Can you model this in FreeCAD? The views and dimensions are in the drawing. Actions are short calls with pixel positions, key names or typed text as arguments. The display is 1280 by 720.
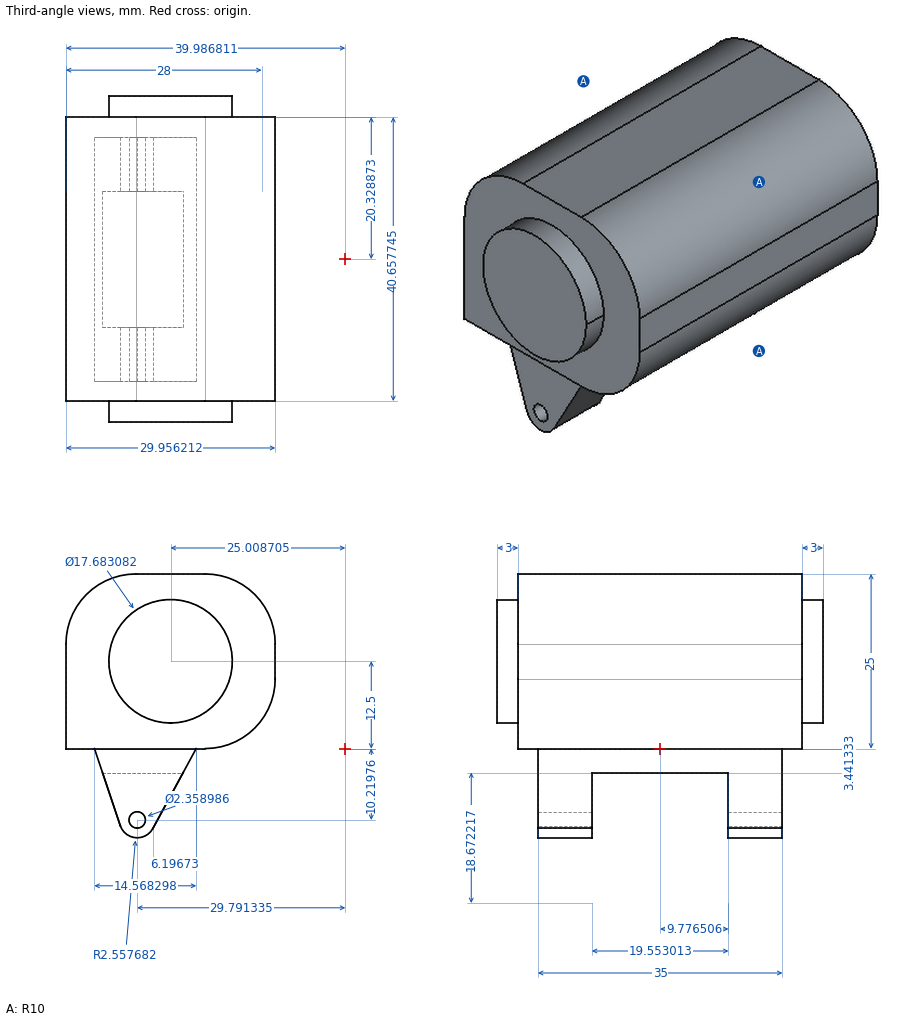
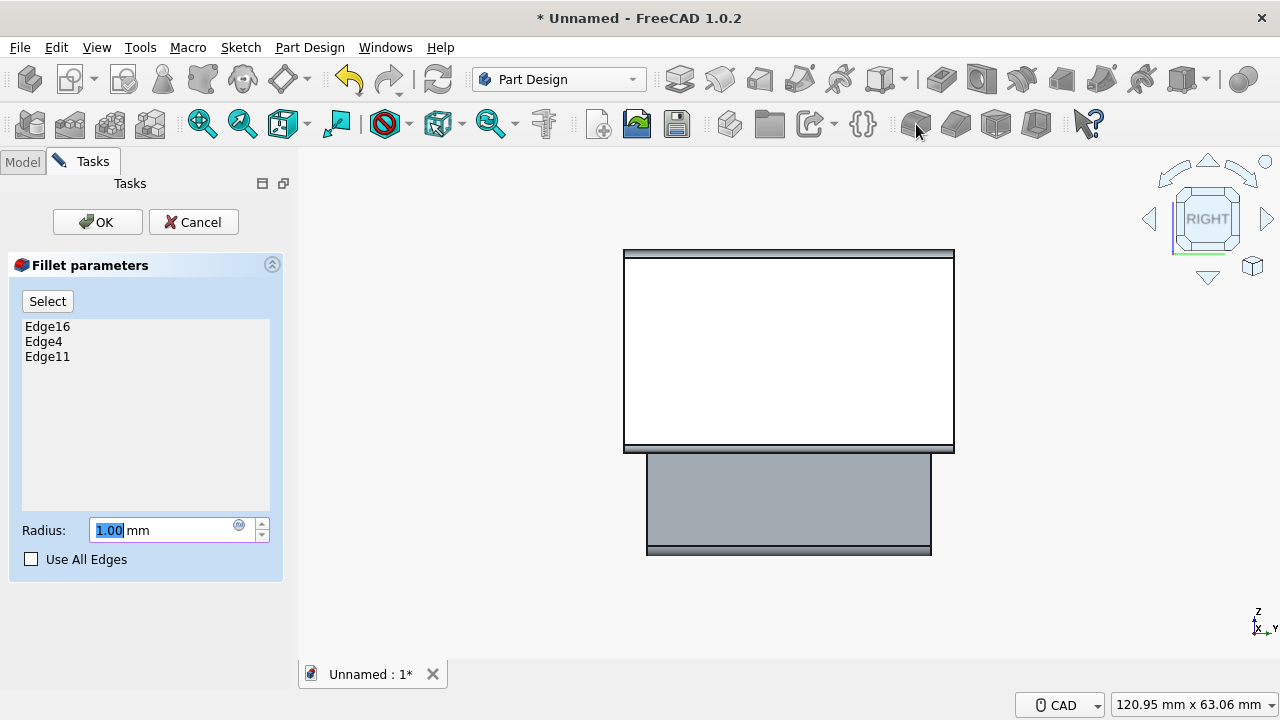
text(10)
key(Tab)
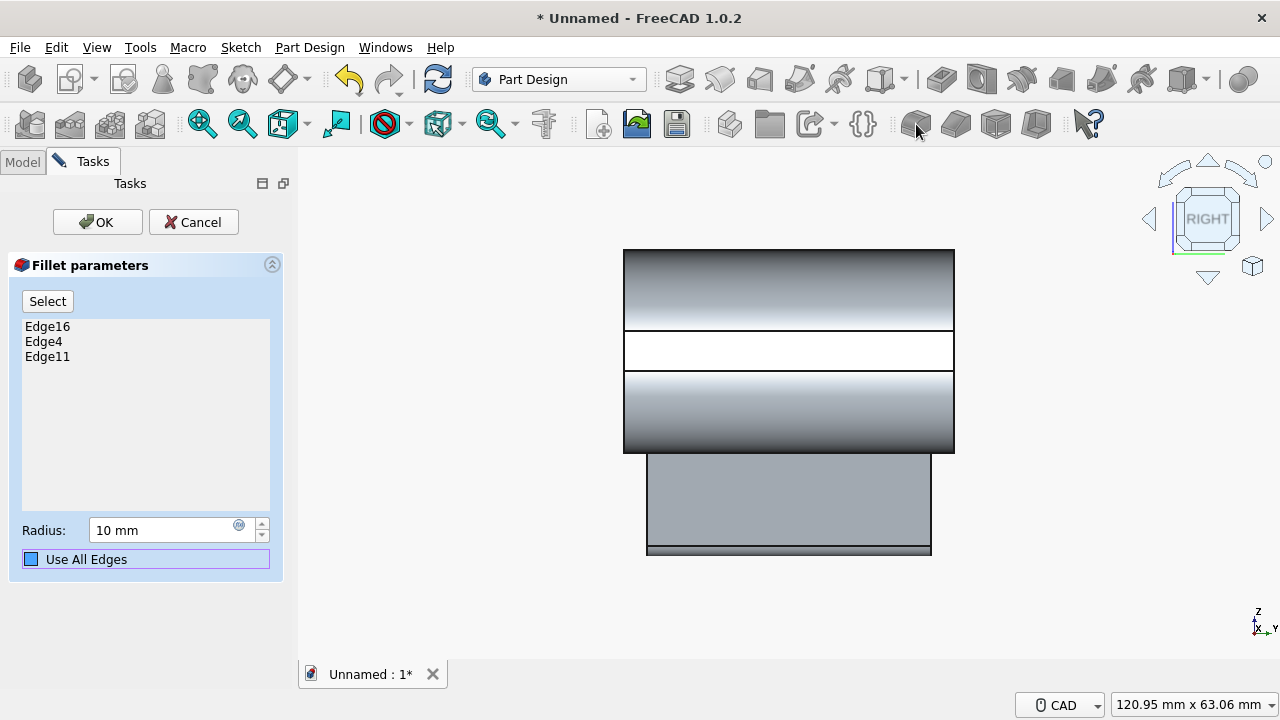
click(98, 222)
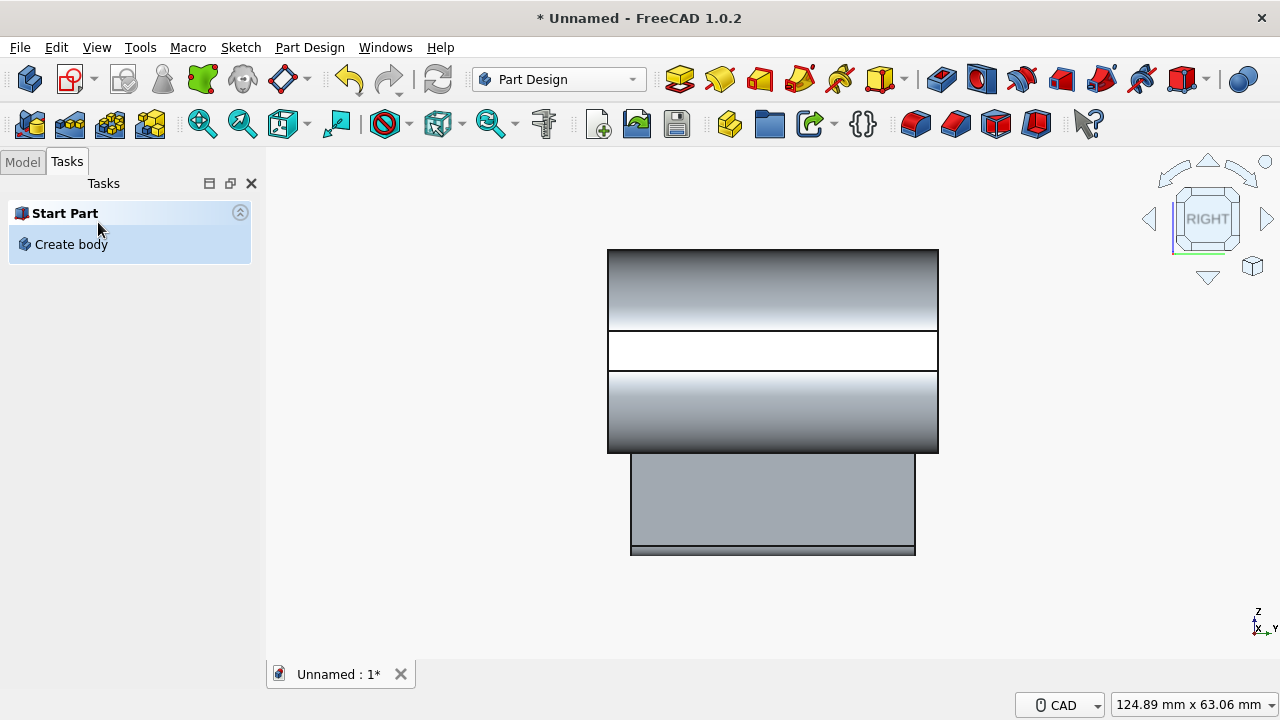
key(0)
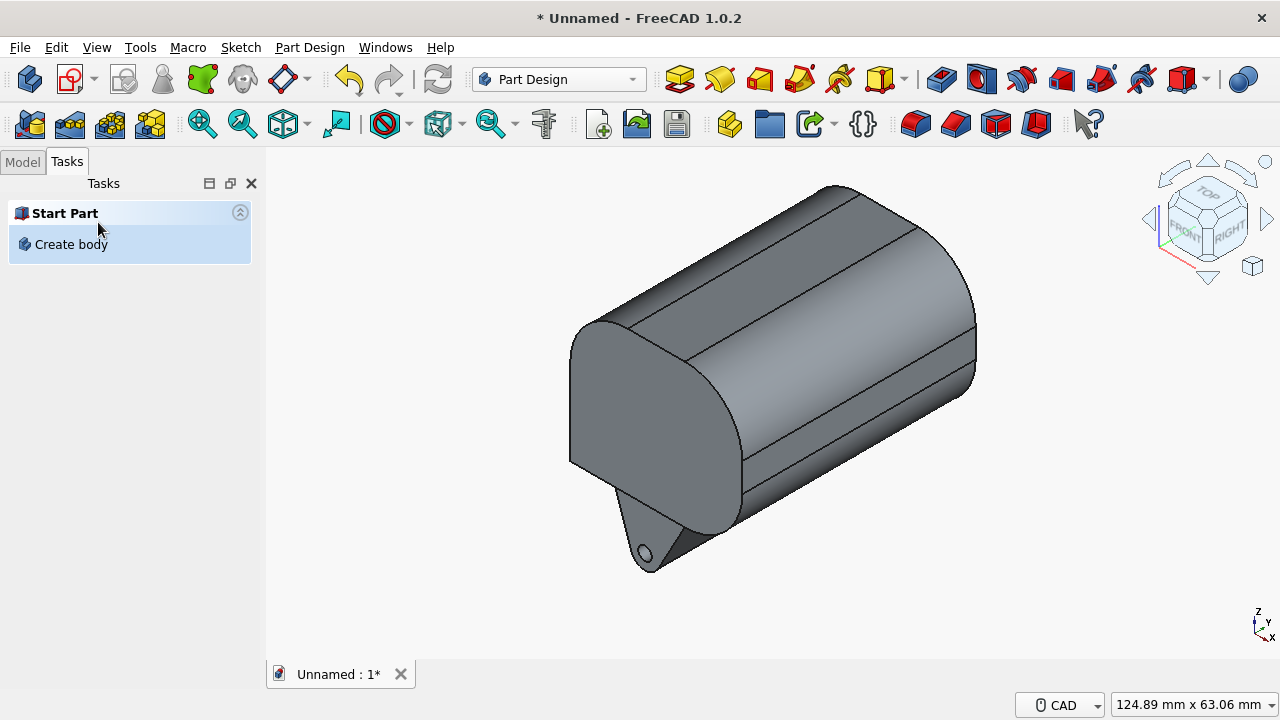
click(656, 427)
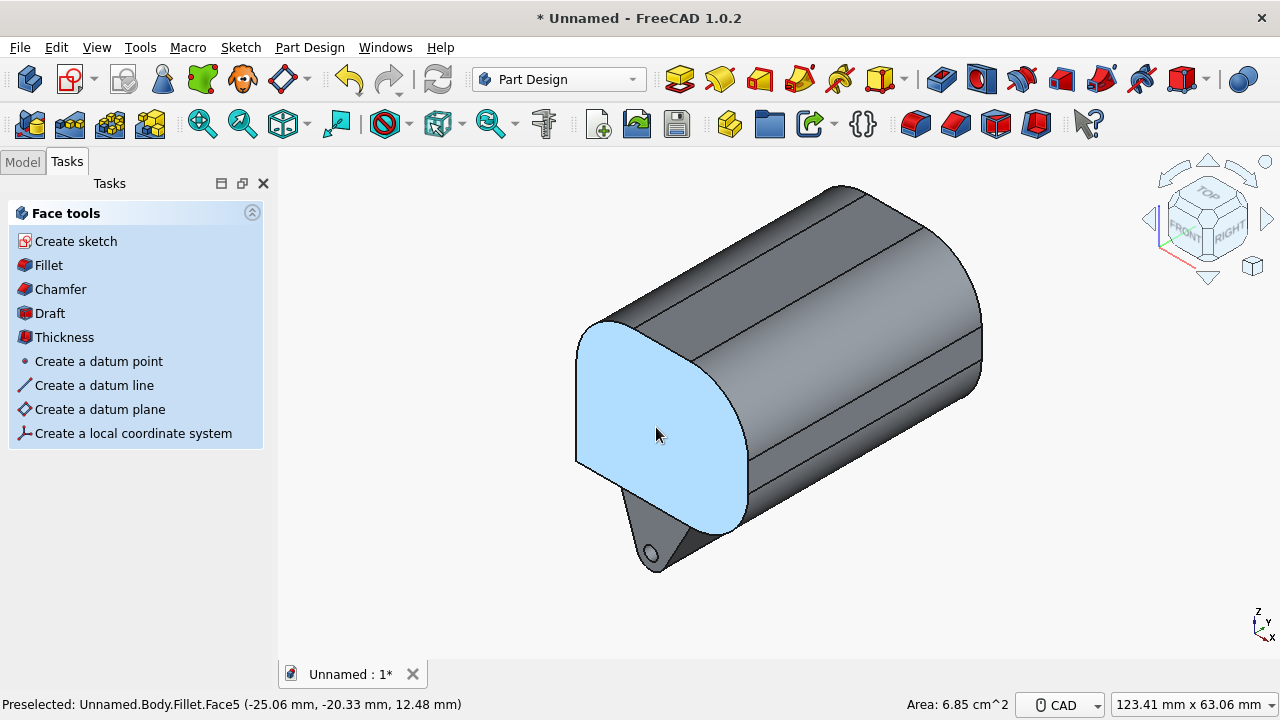
click(70, 80)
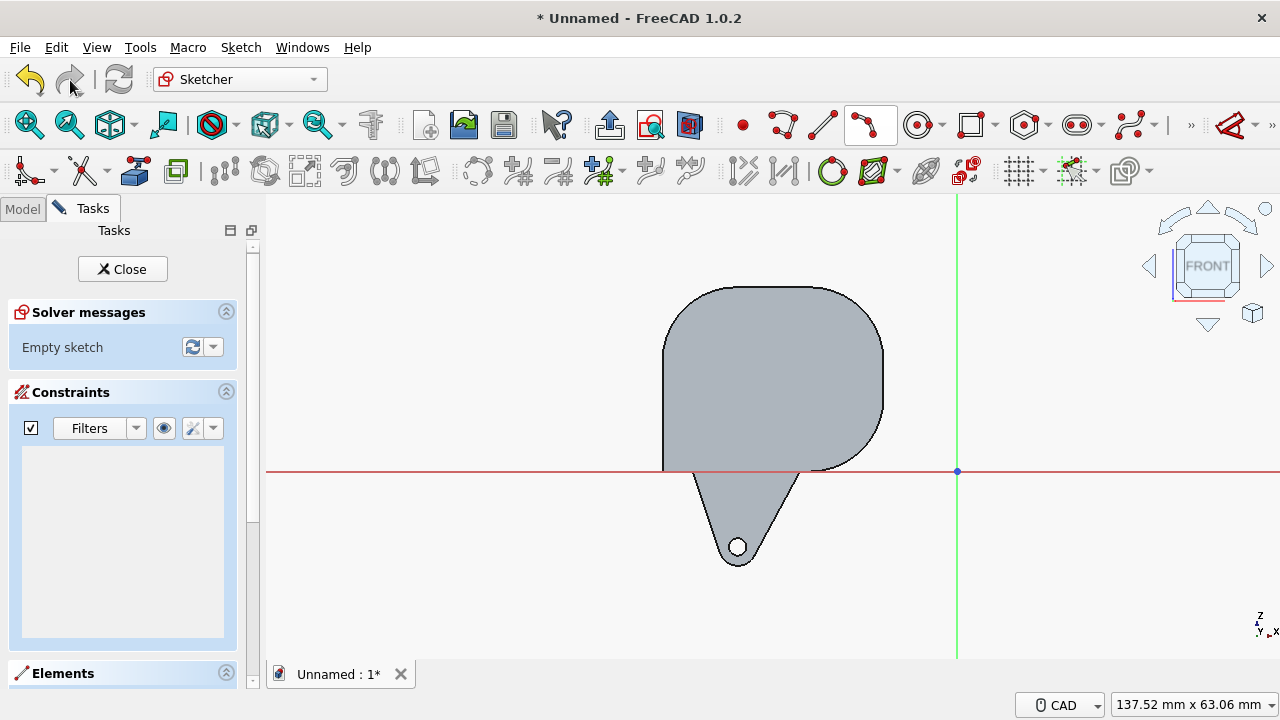
scroll(988, 352, up, 3)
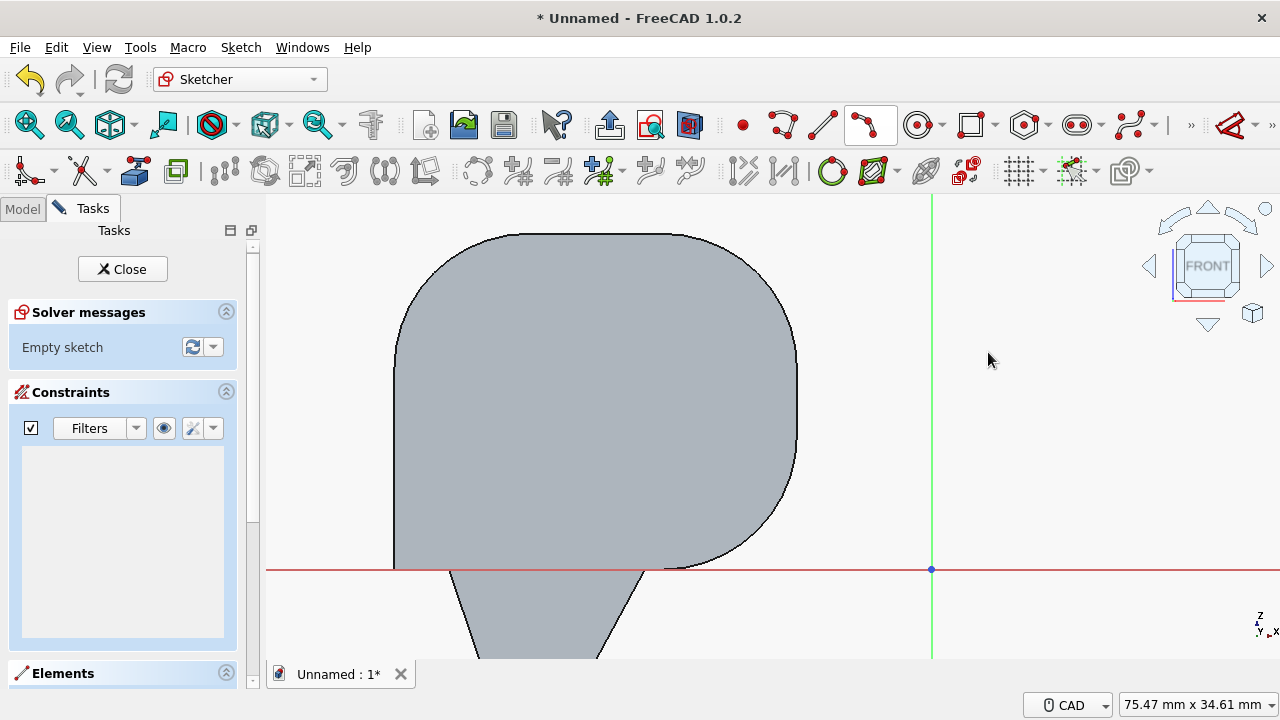
click(918, 126)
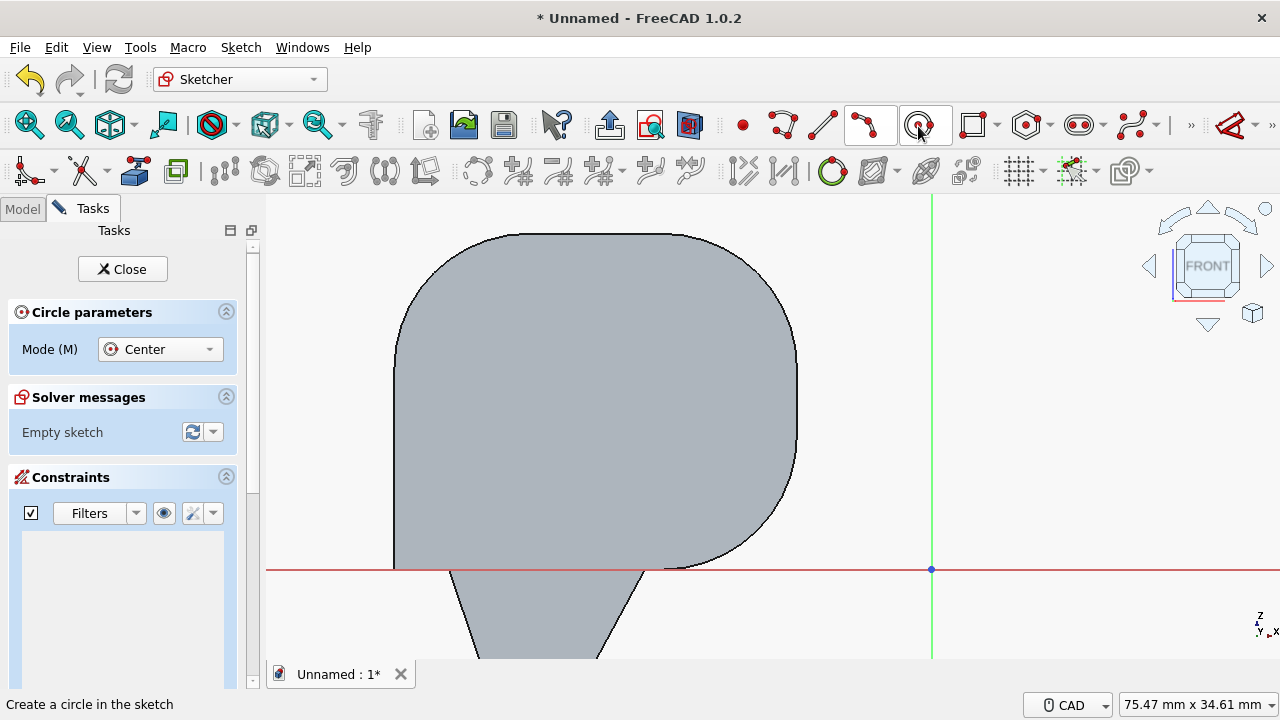
click(596, 402)
move(680, 318)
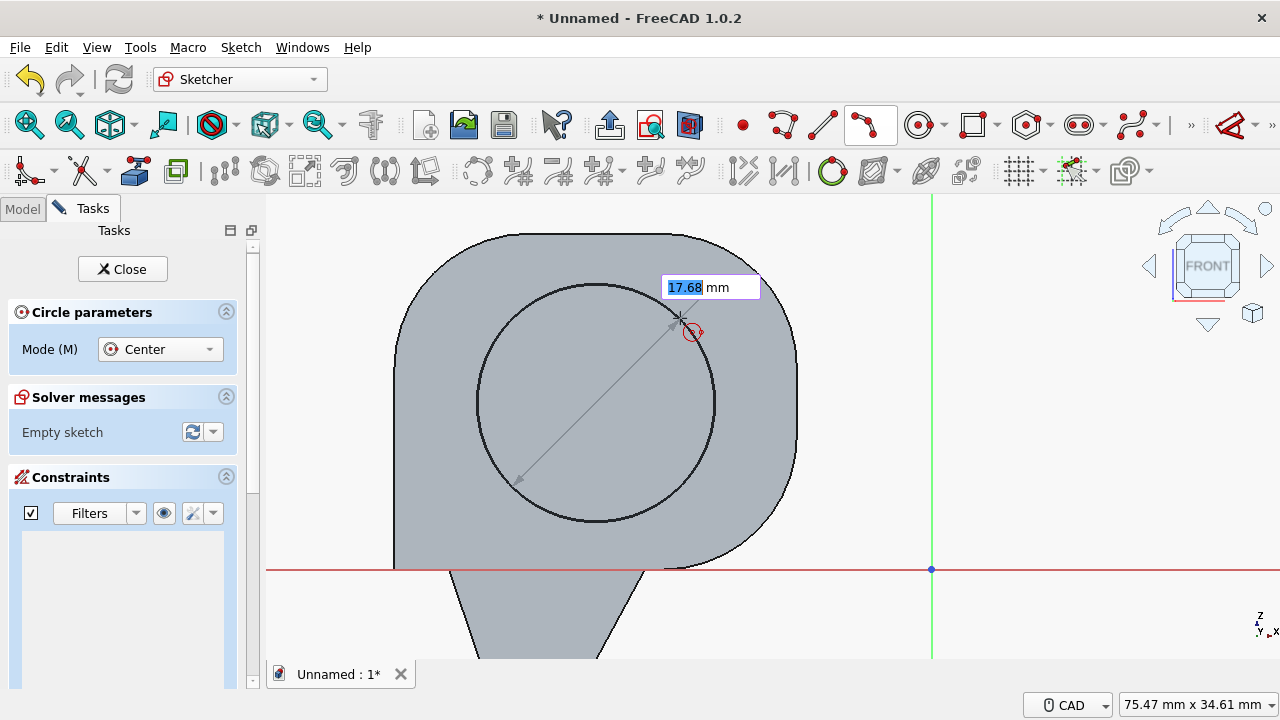
text(17.683082)
key(Return)
key(Escape)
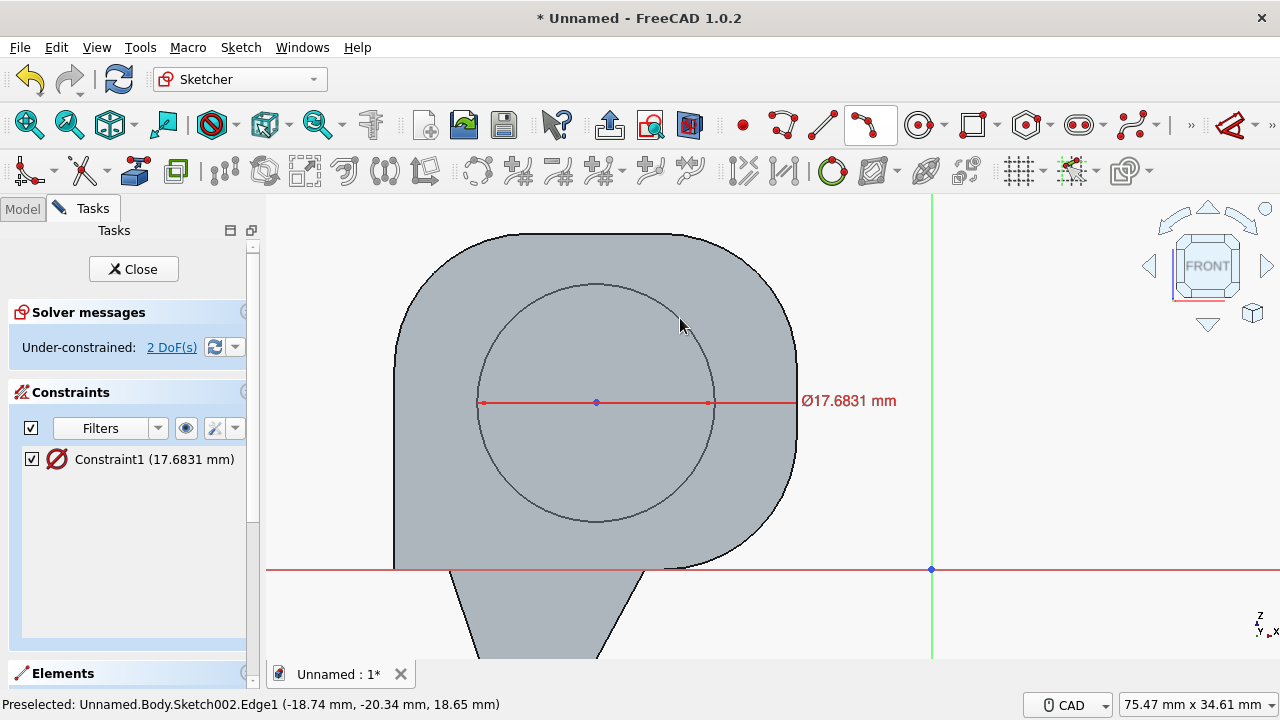
click(1230, 126)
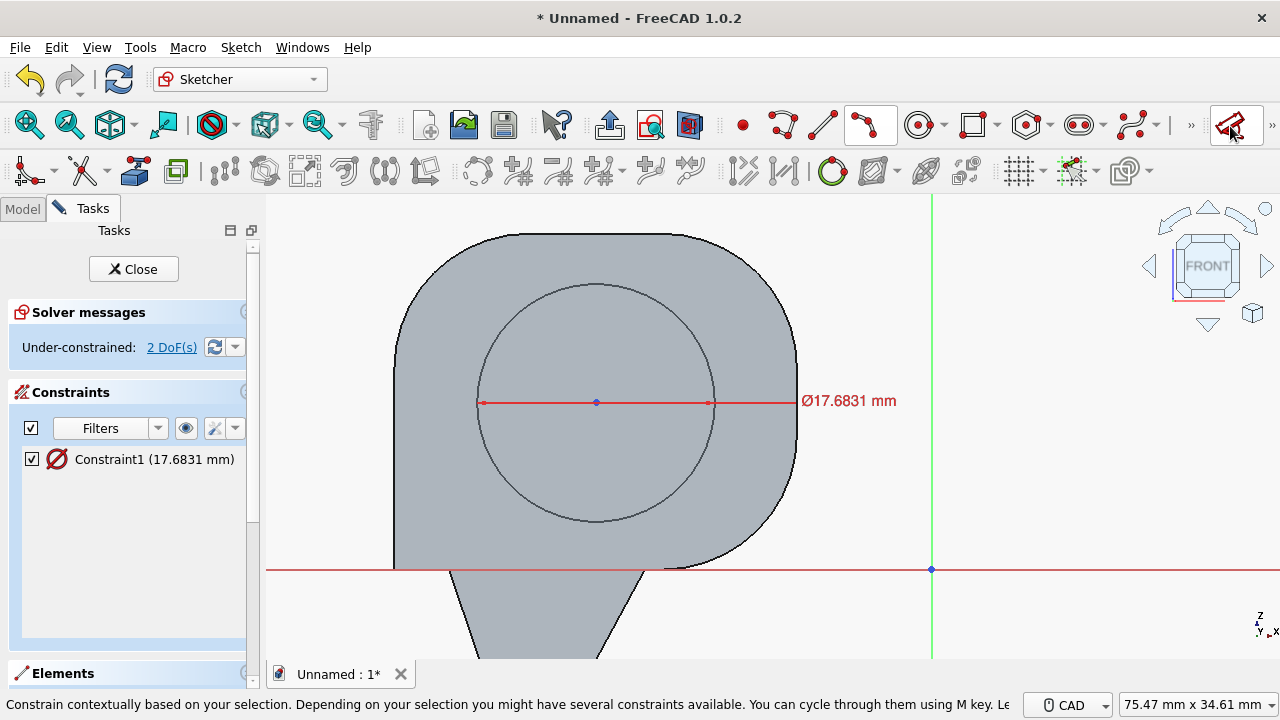
click(596, 403)
click(966, 486)